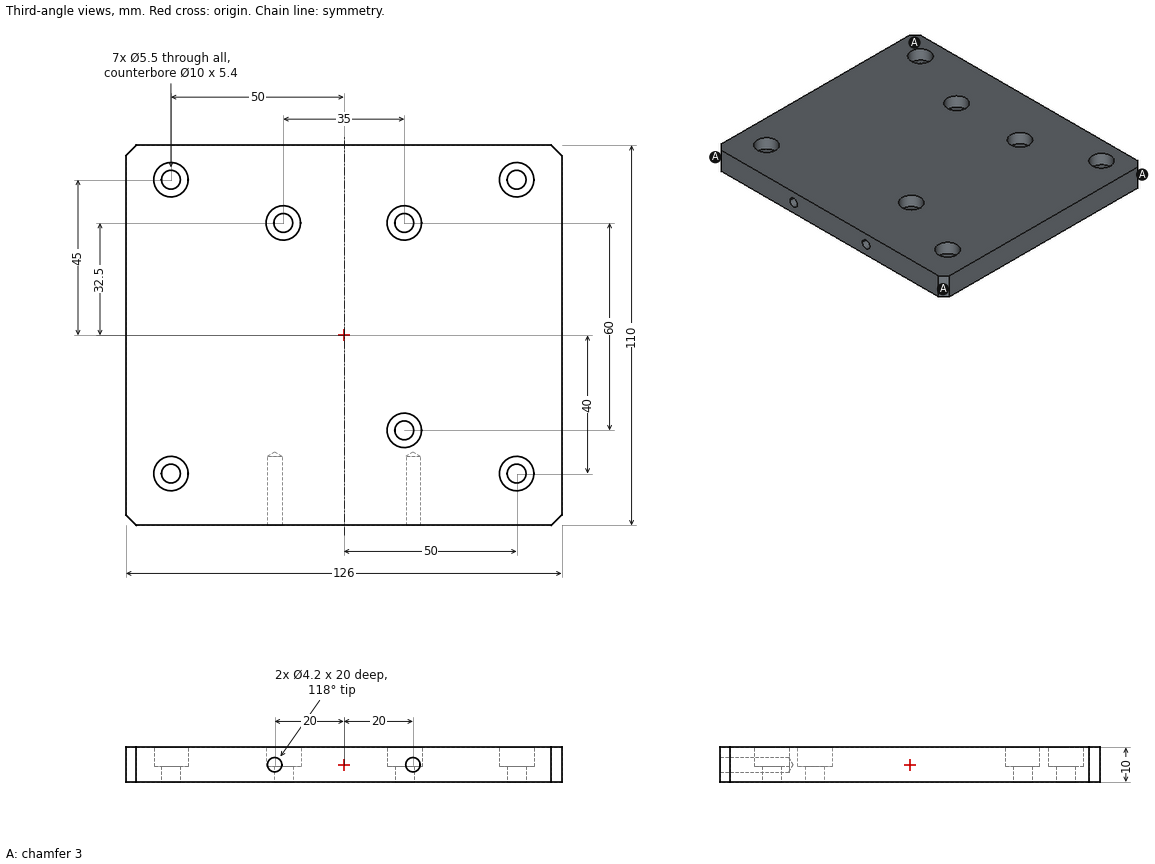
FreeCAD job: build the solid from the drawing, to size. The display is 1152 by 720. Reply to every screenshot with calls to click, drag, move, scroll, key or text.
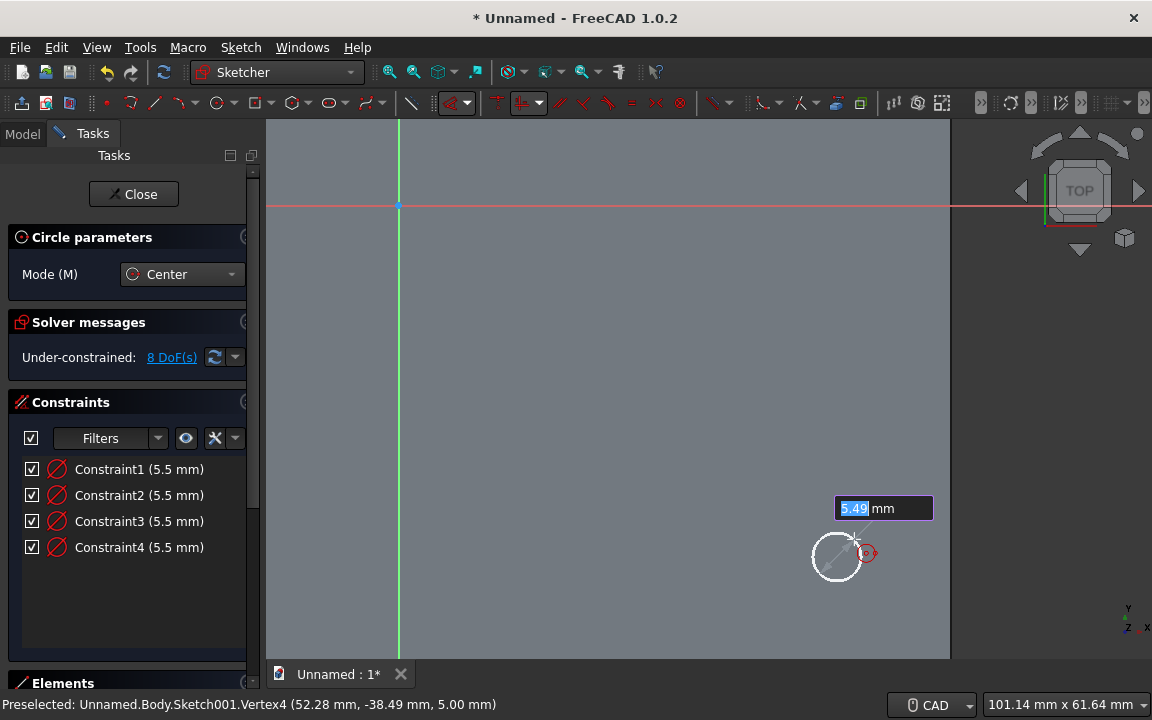
text(5.5)
key(Return)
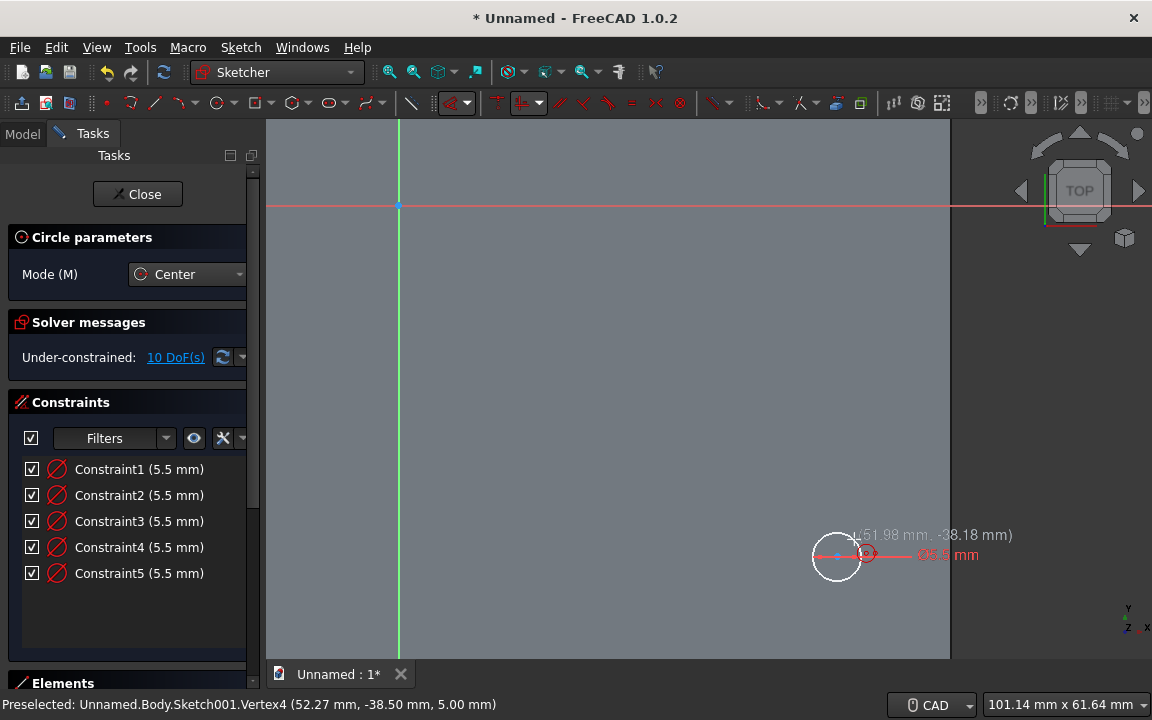
click(552, 446)
move(569, 429)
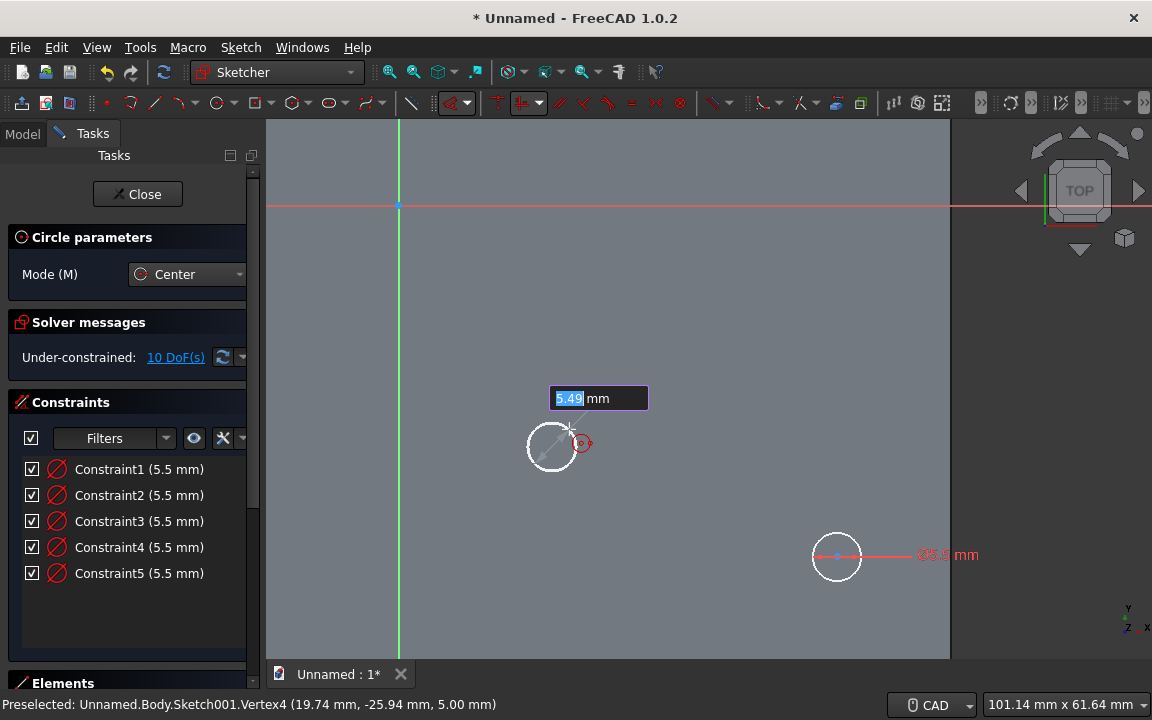
text(5.5)
key(Return)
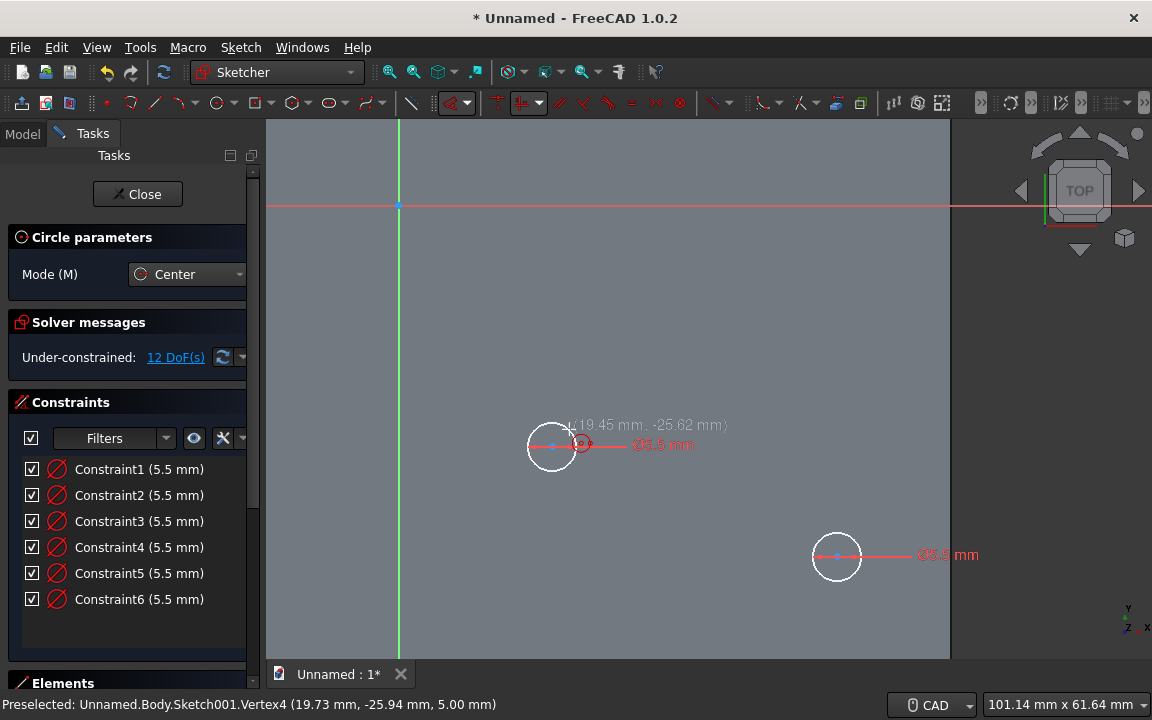
scroll(838, 557, down, 4)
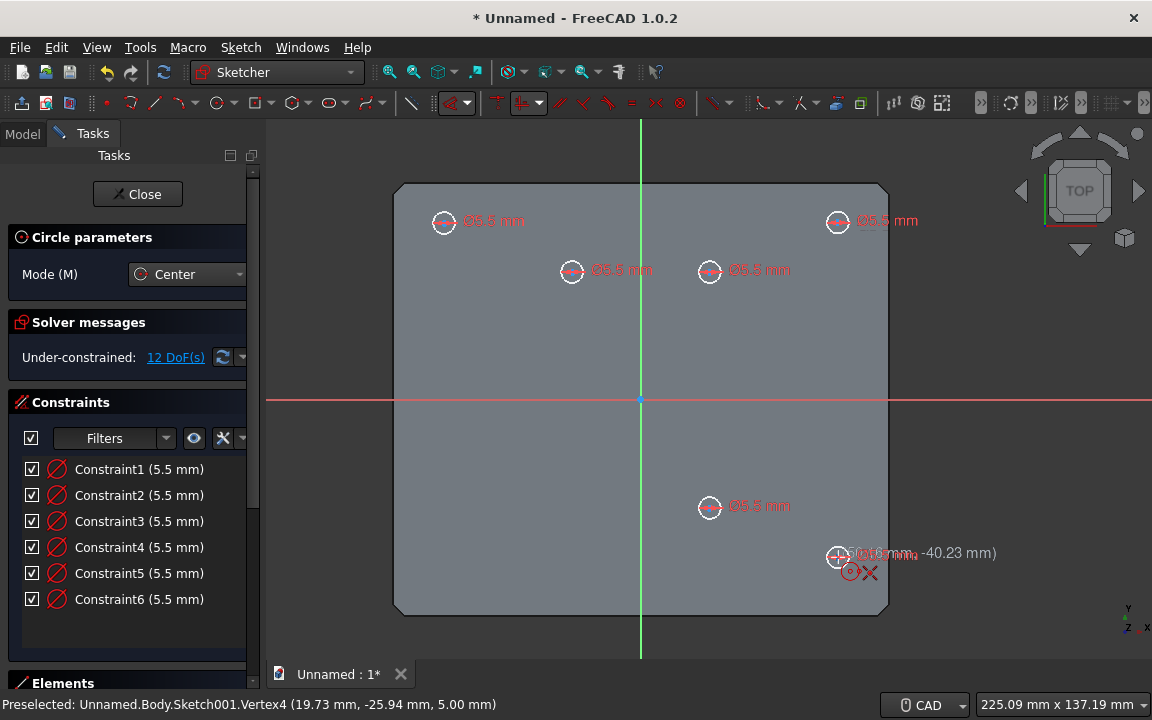
scroll(444, 557, up, 4)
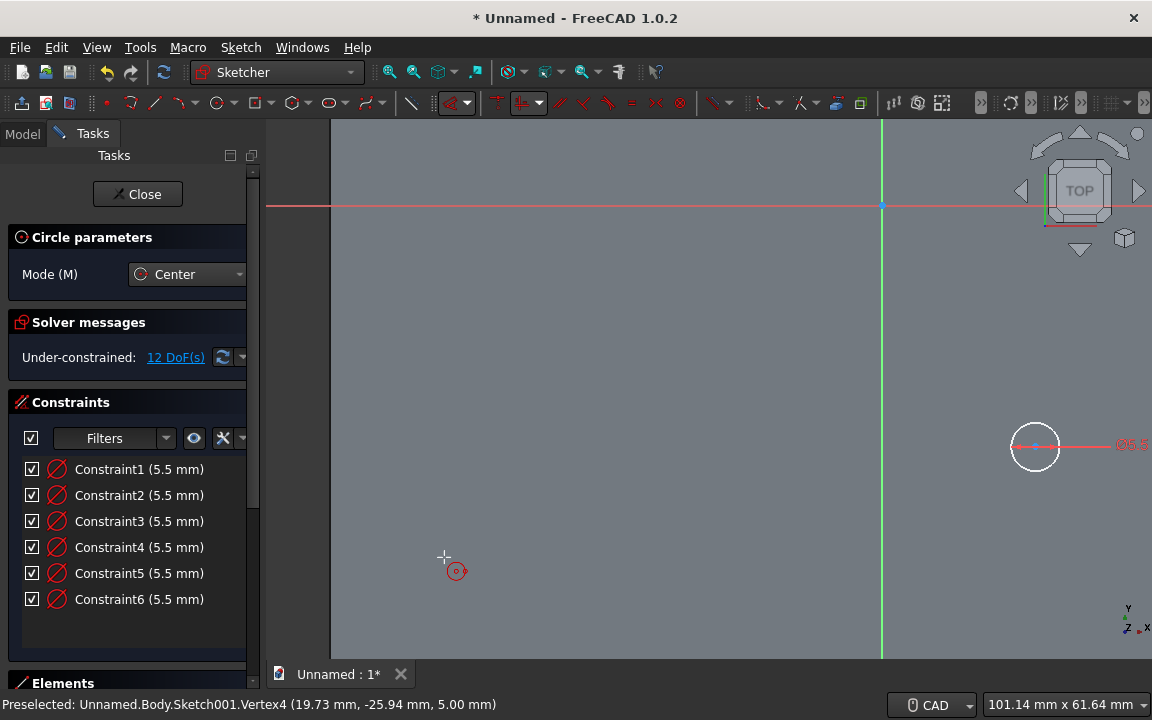
click(444, 556)
move(461, 539)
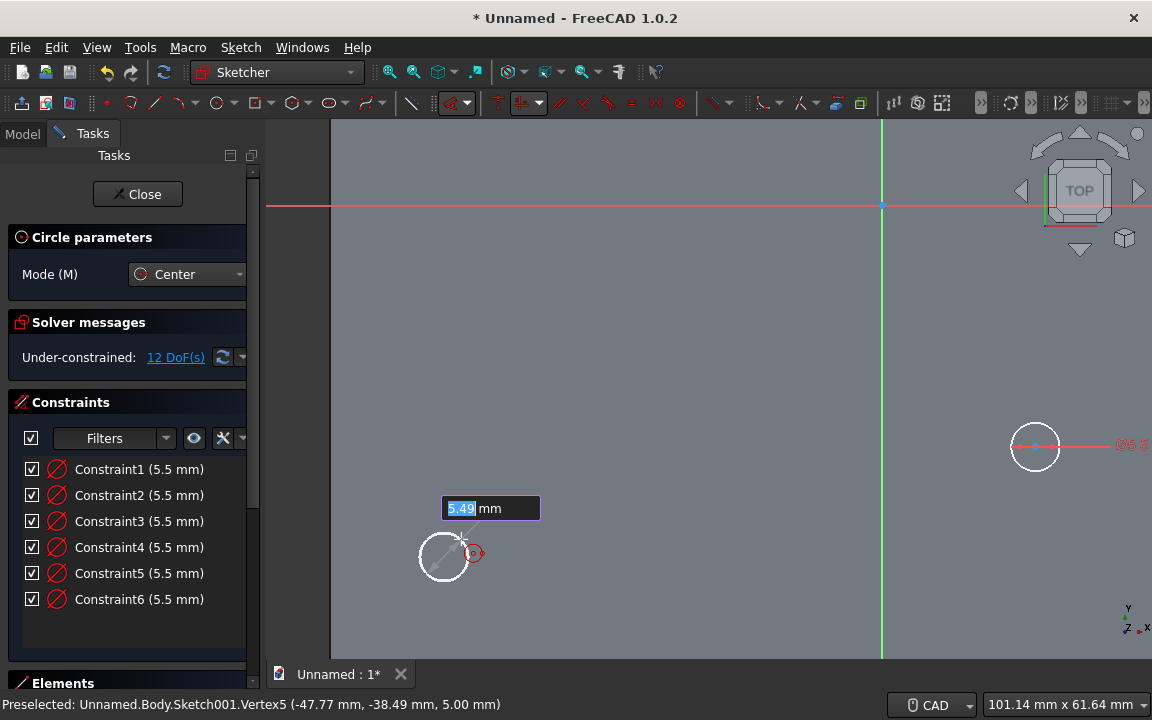
text(5.5)
key(Return)
key(Escape)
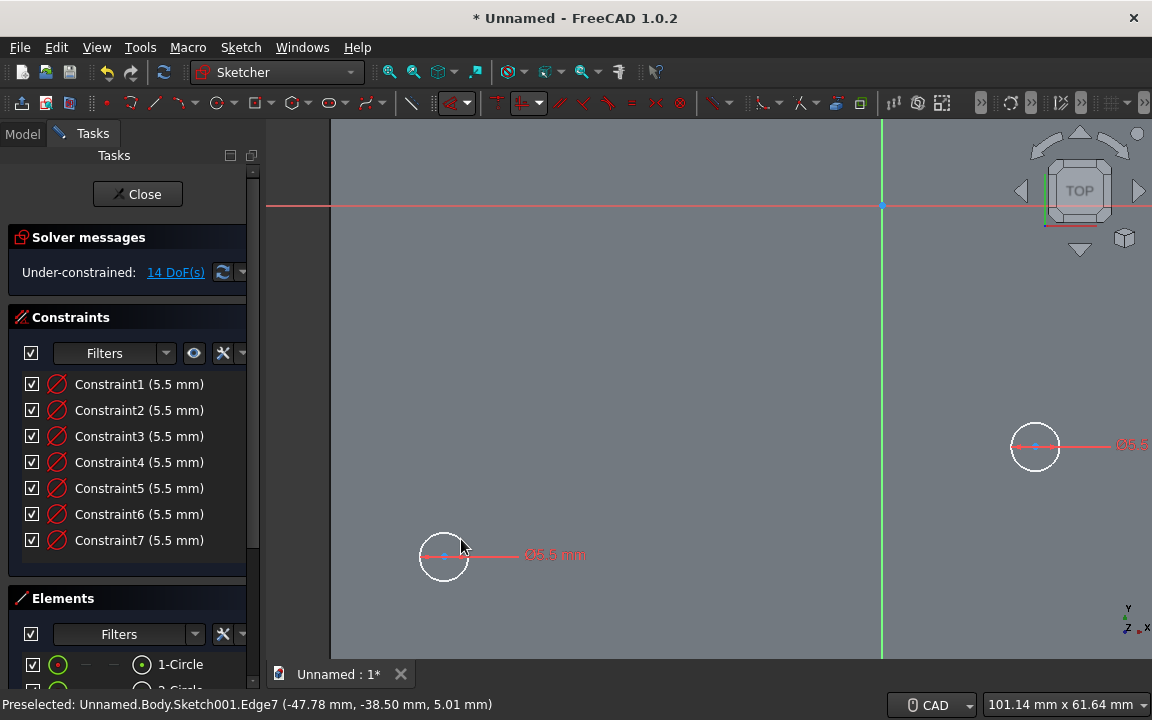
scroll(443, 557, down, 4)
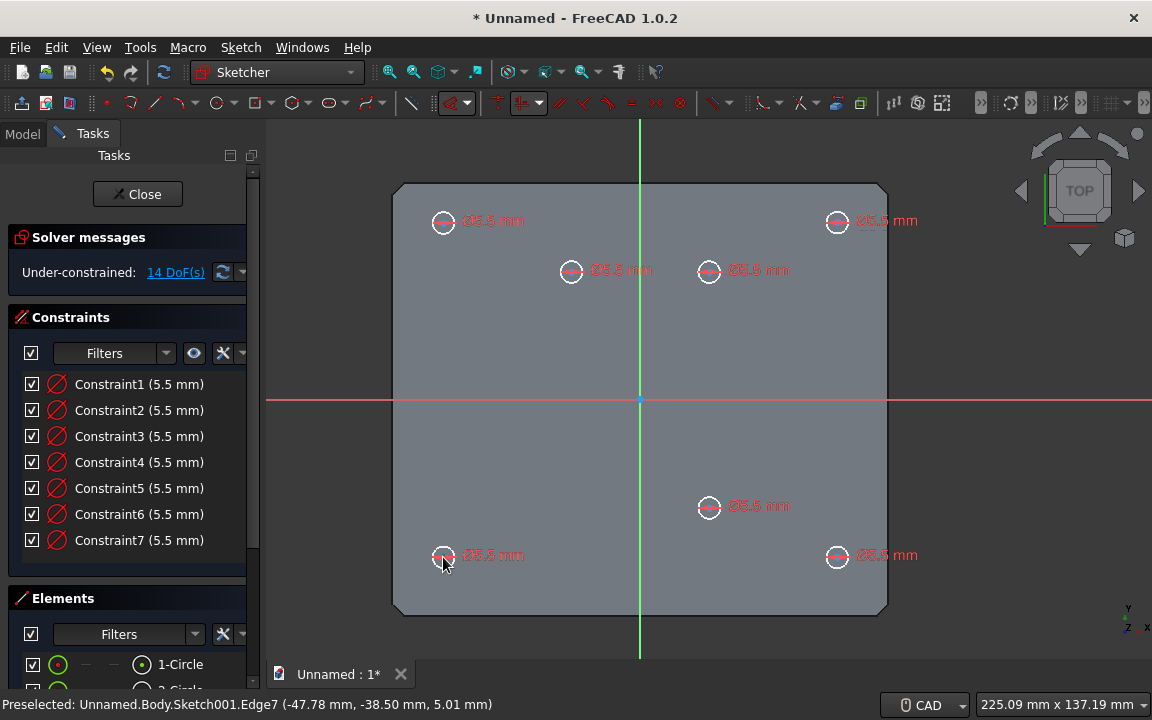
click(572, 272)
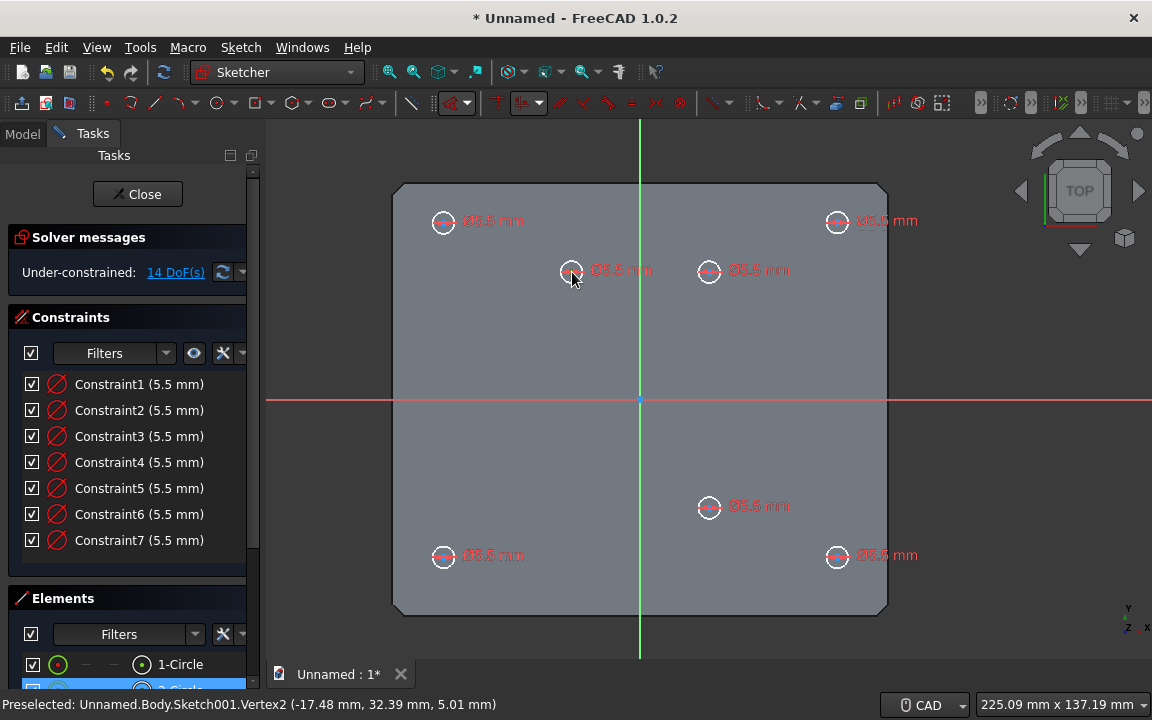
click(709, 272)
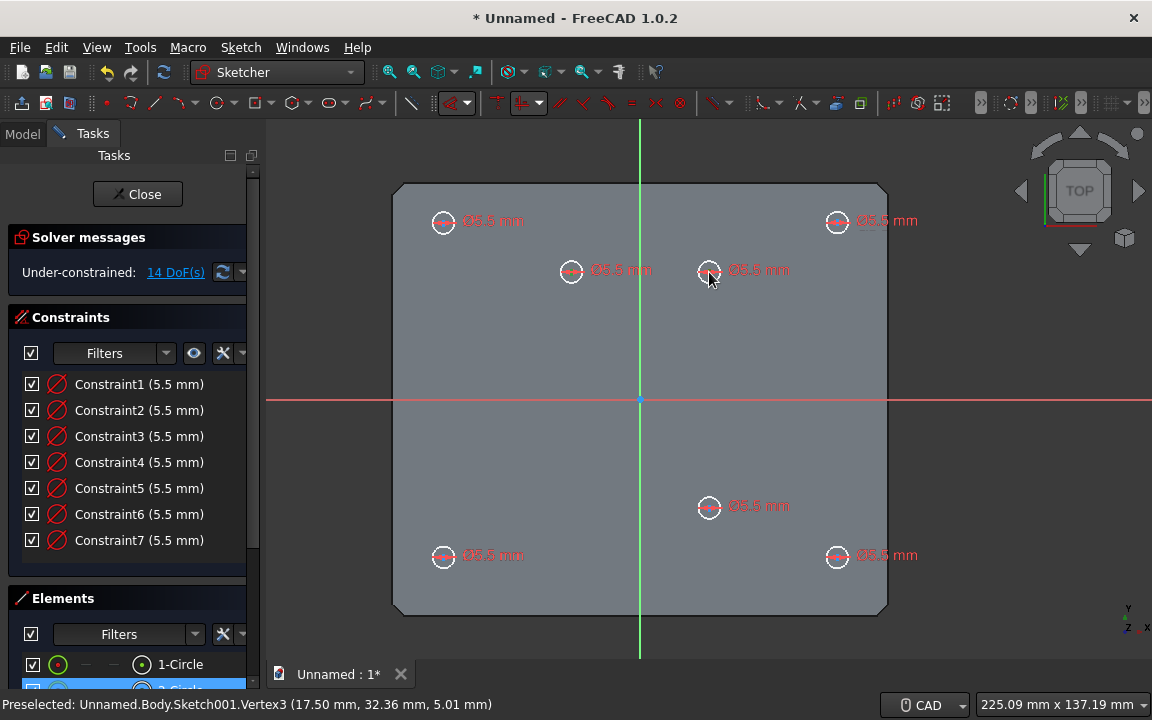
click(640, 596)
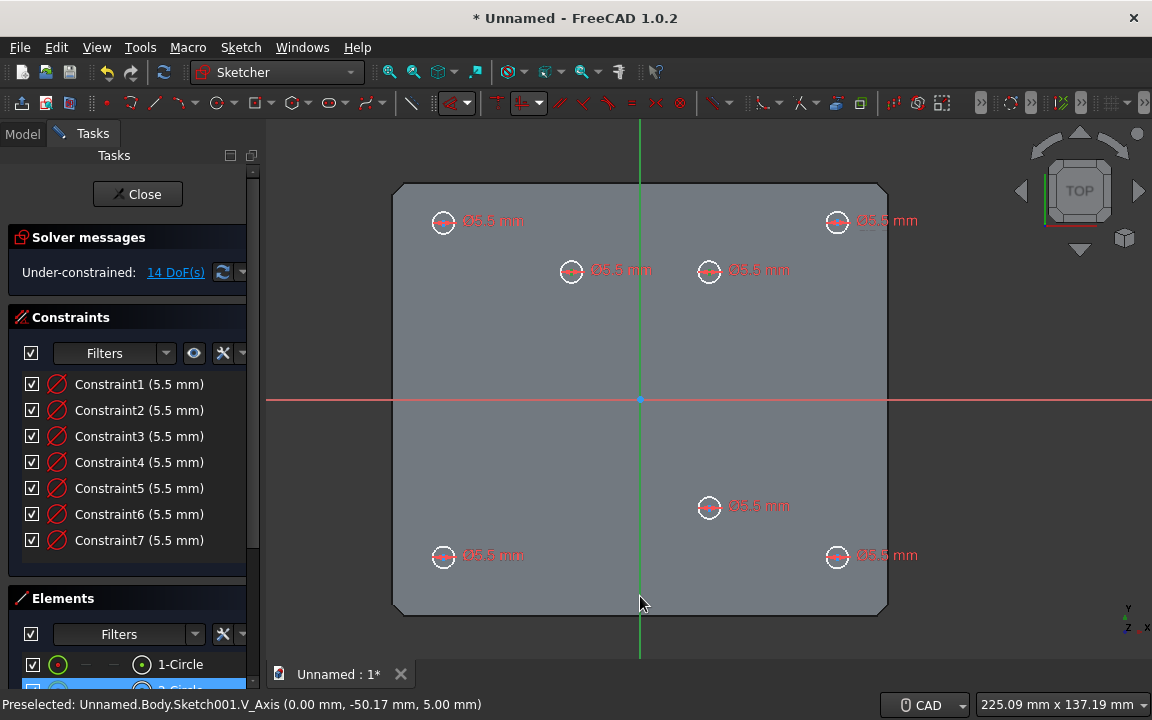
click(656, 104)